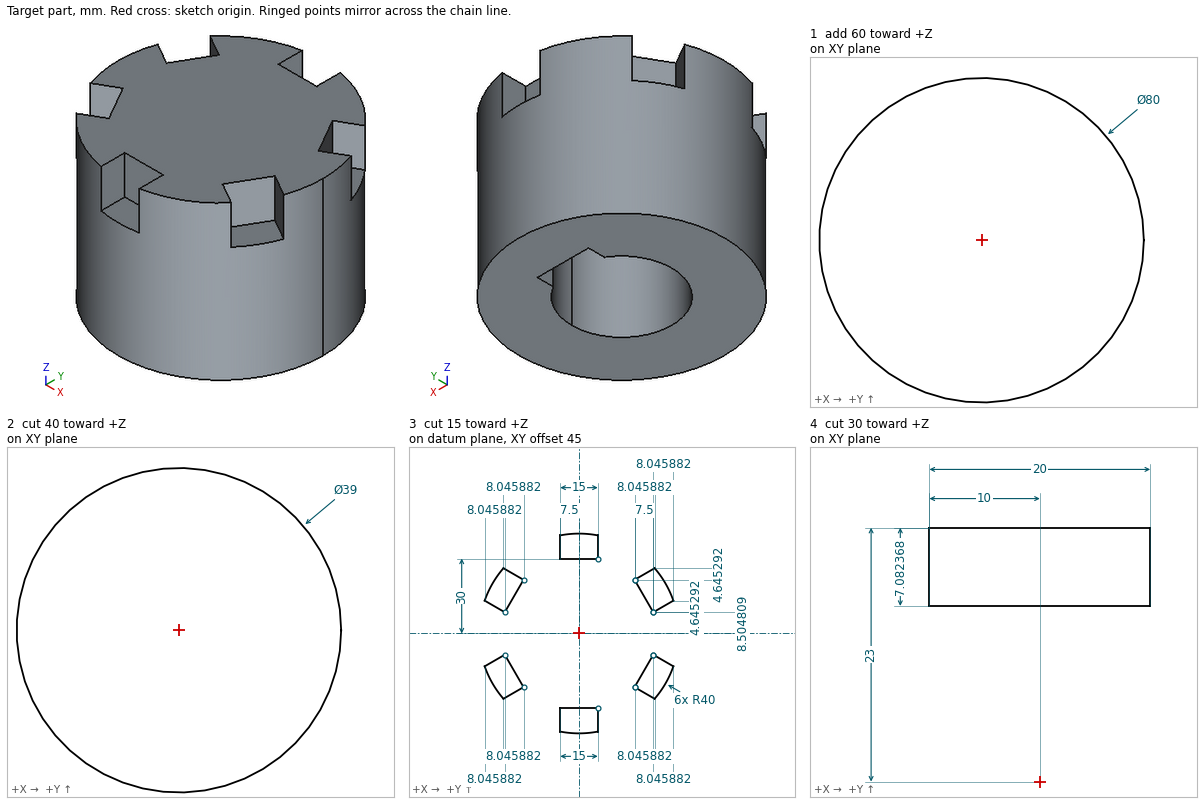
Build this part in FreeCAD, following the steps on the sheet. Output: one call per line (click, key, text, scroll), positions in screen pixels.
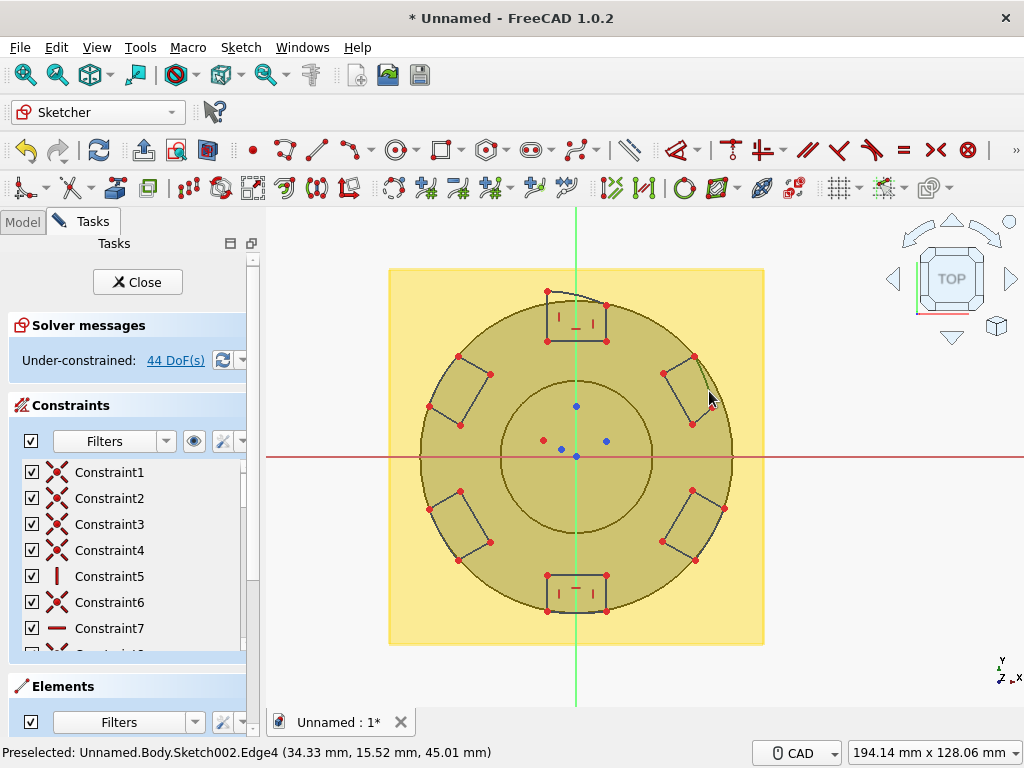
click(565, 613)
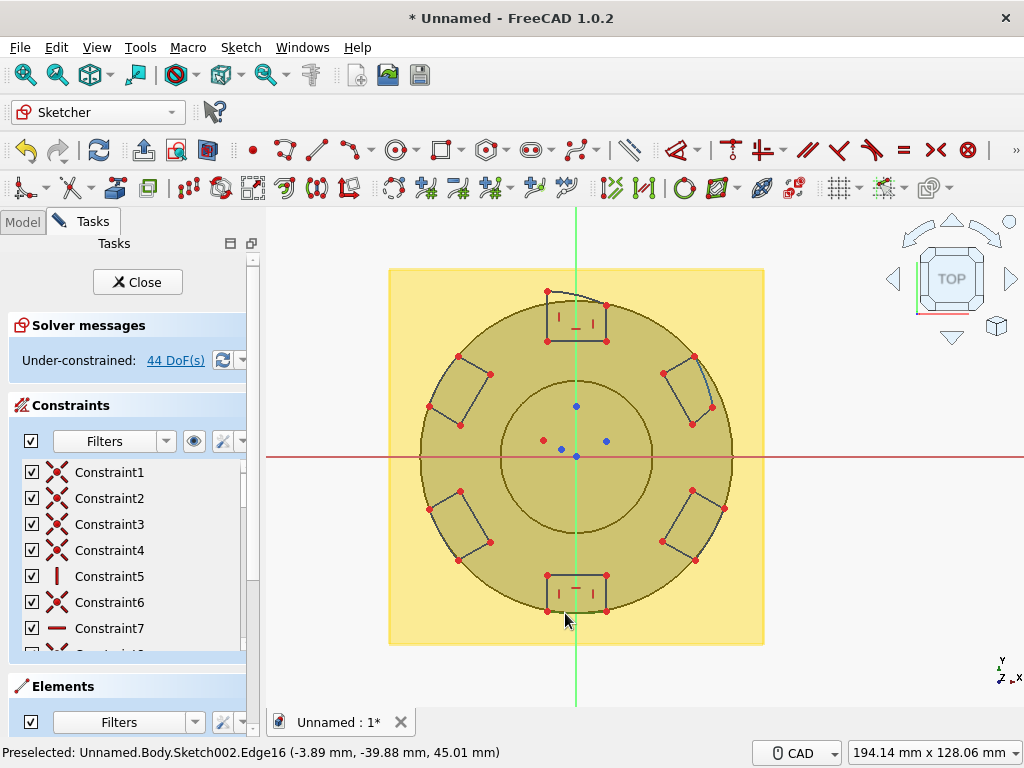
click(732, 150)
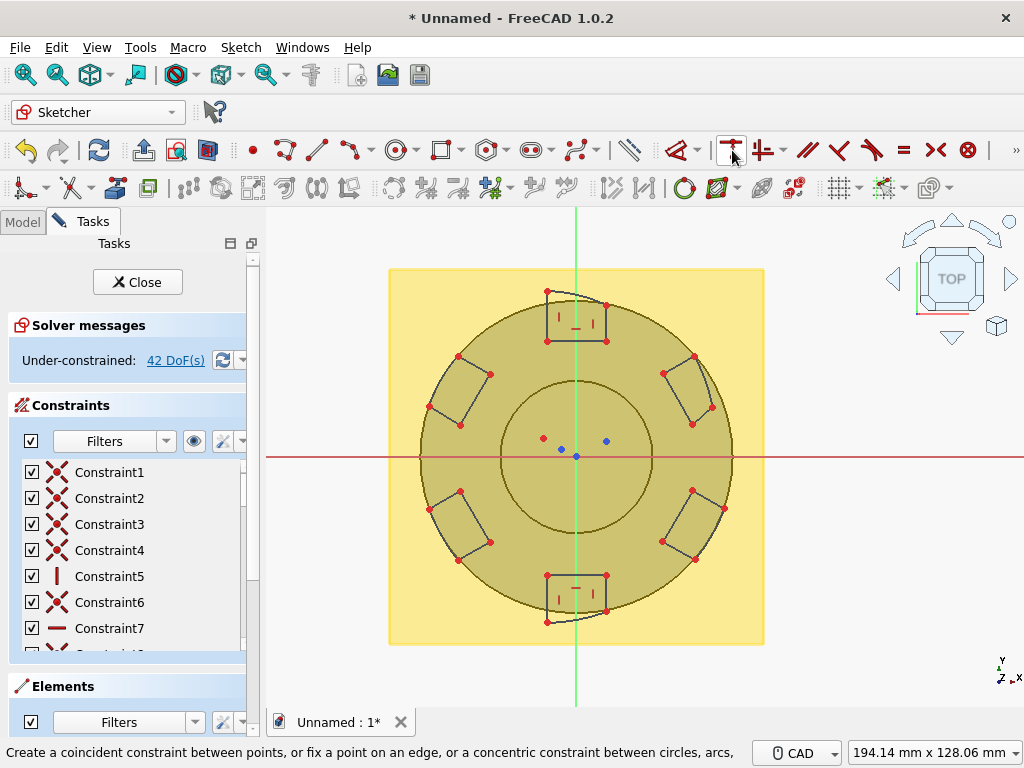
click(709, 391)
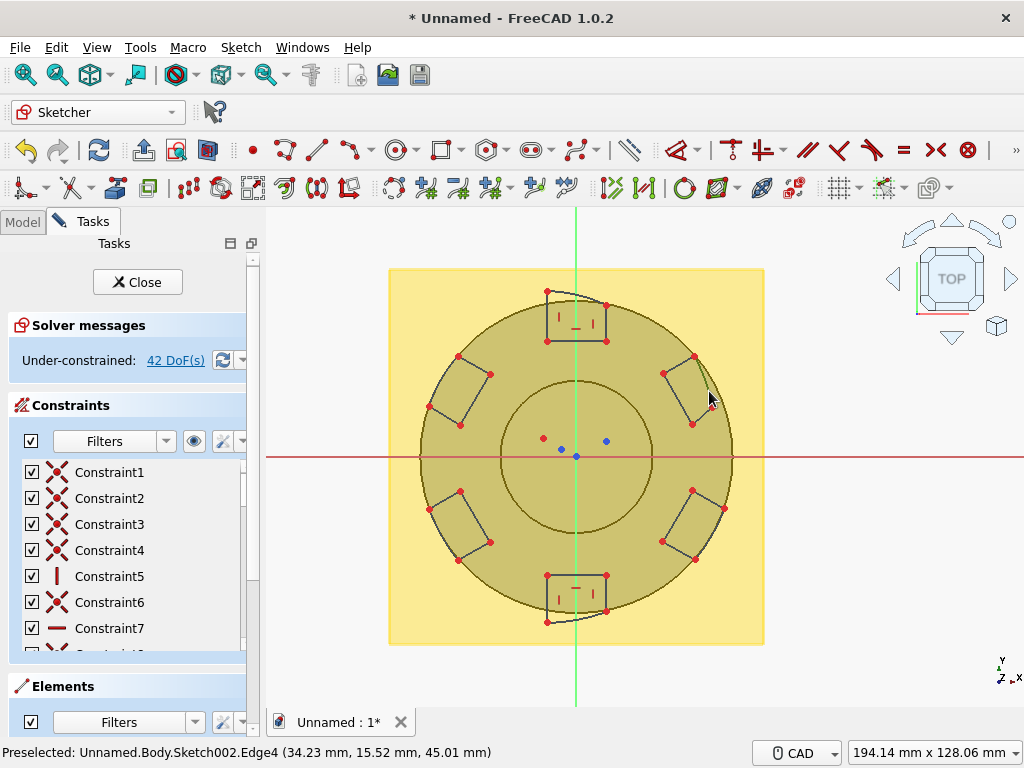
click(436, 525)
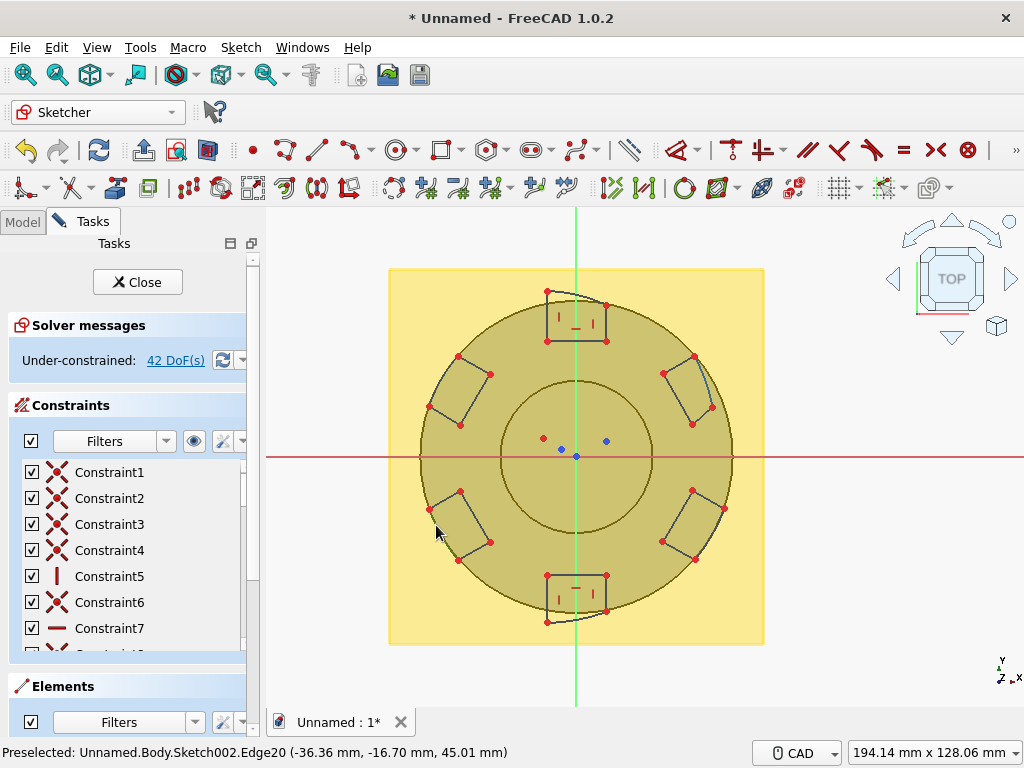
click(732, 150)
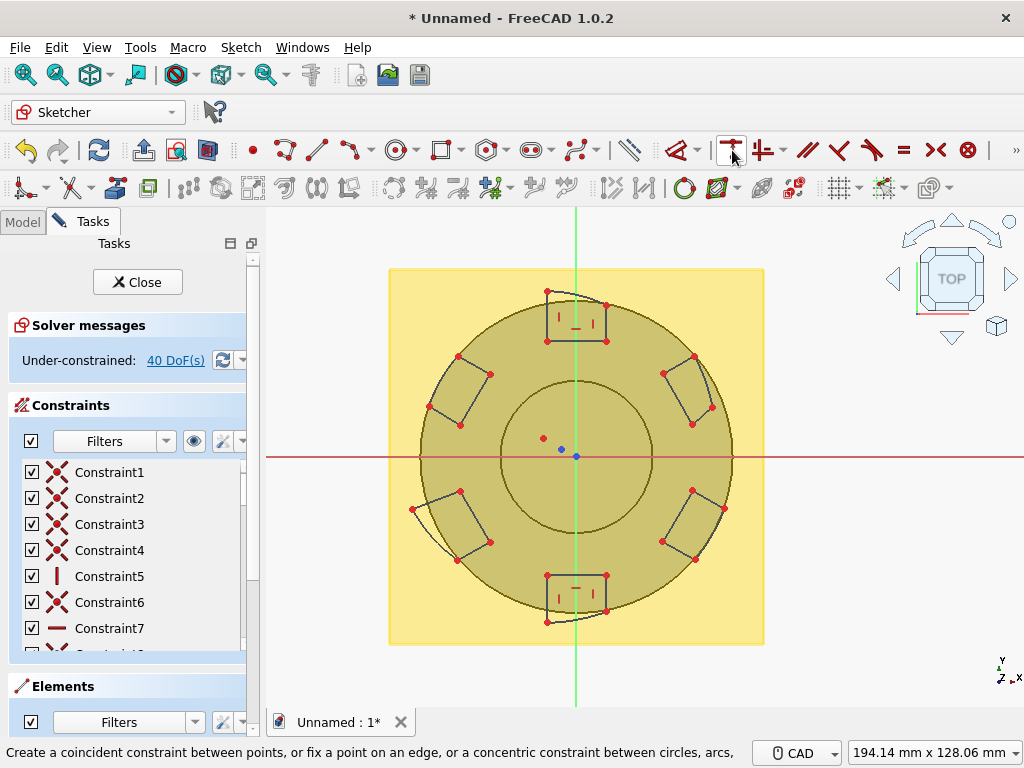
click(709, 391)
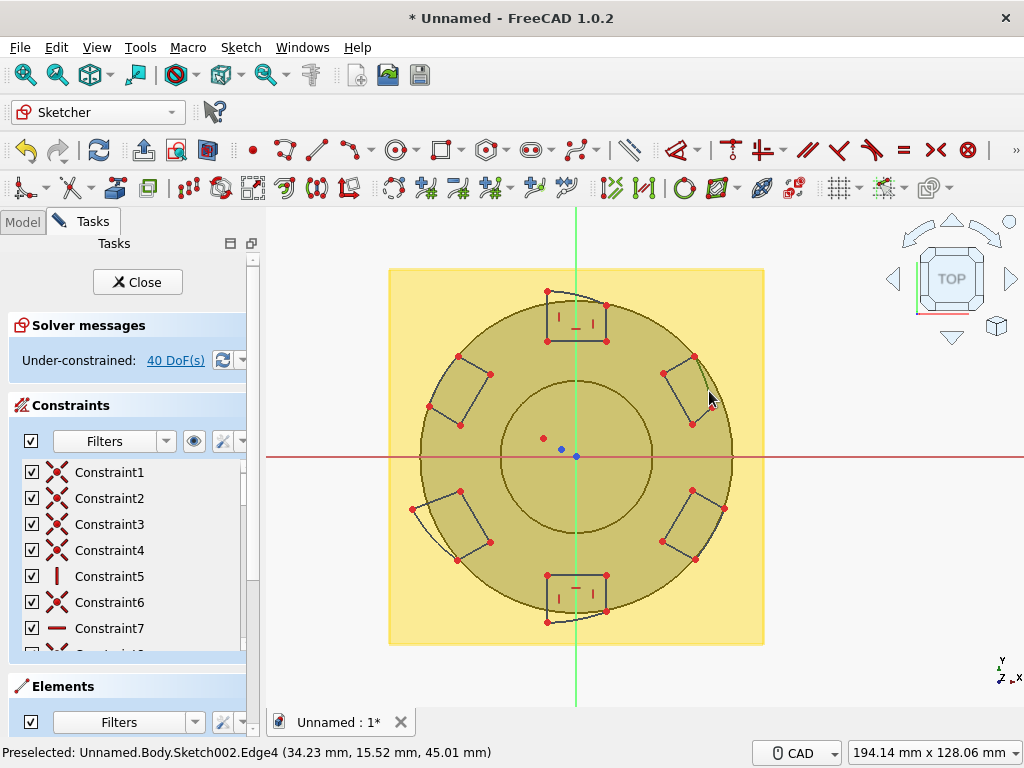
click(447, 370)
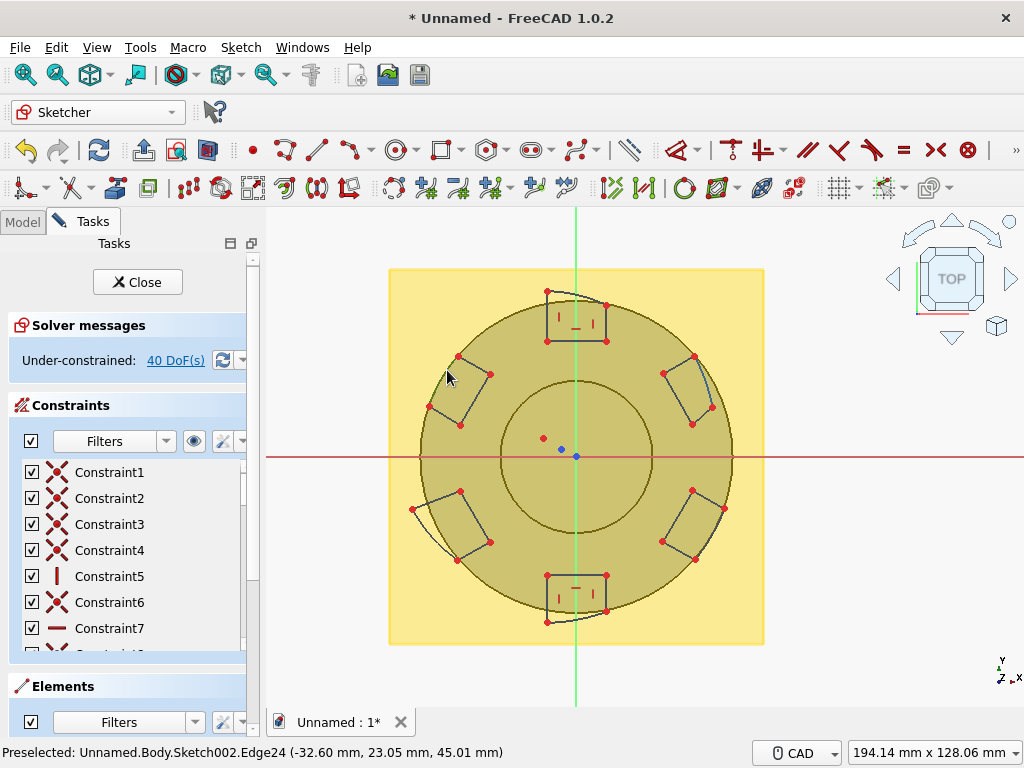
key(c)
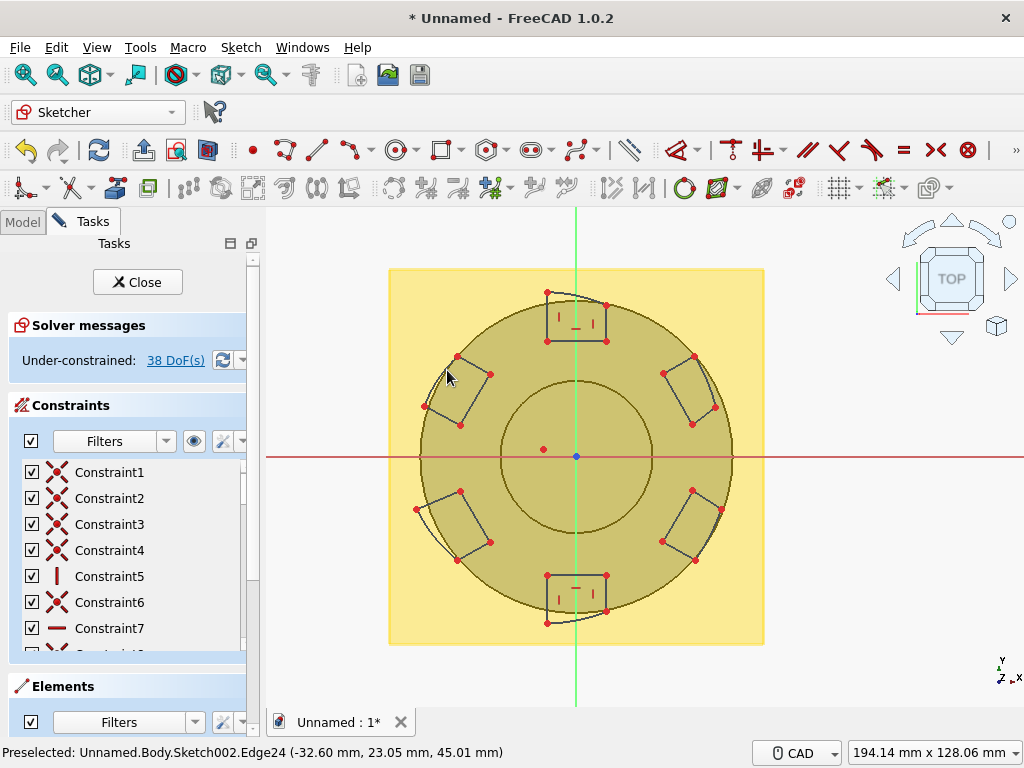
drag(534, 440, 586, 467)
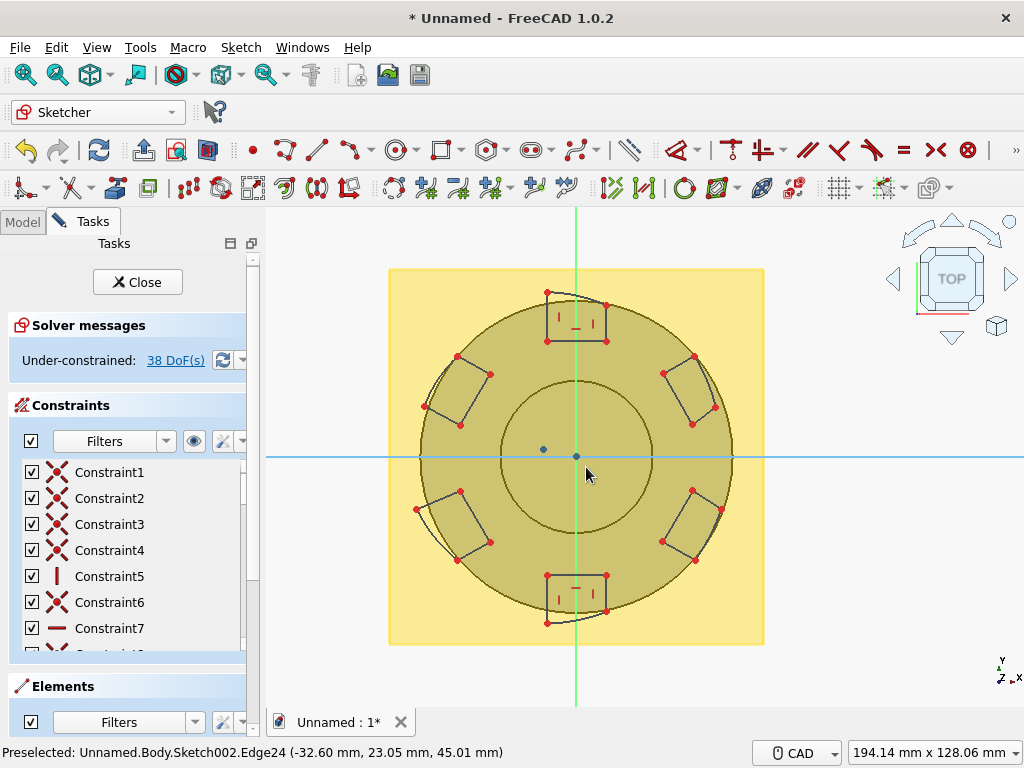
click(732, 150)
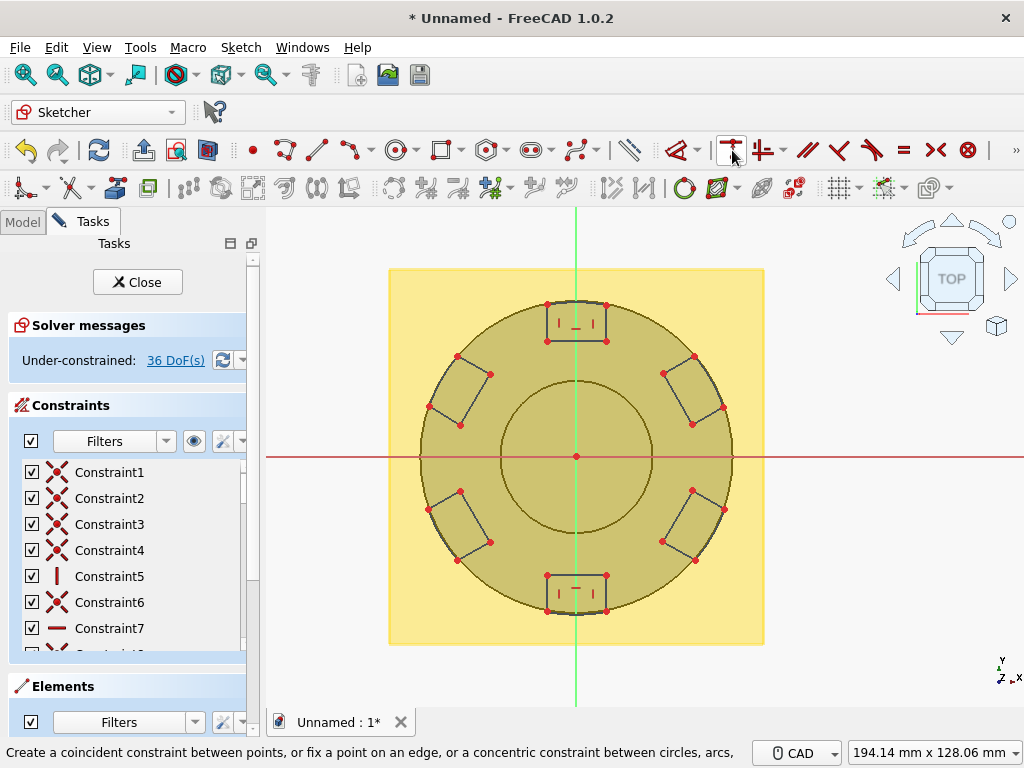
click(717, 391)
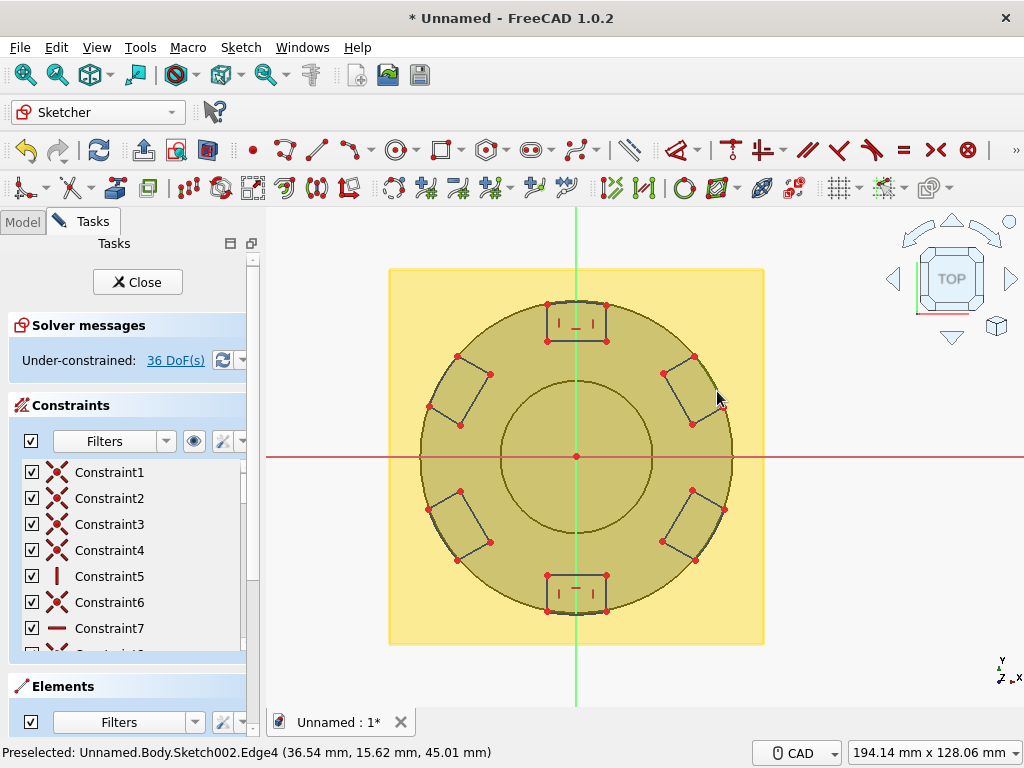
click(588, 303)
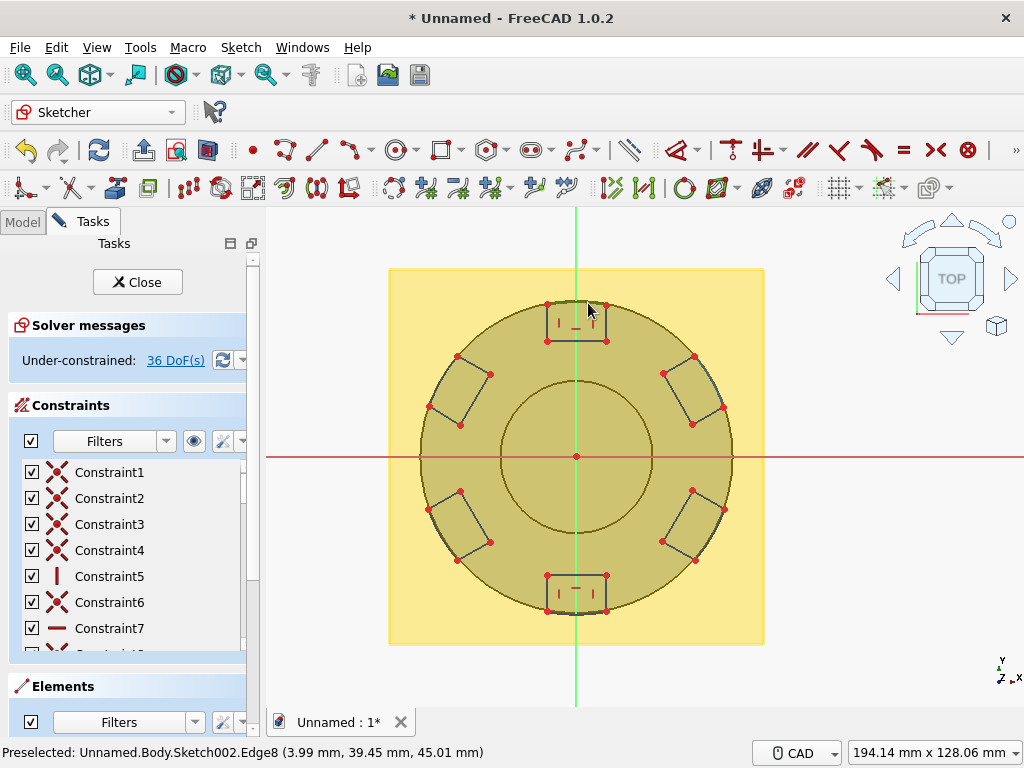
click(706, 546)